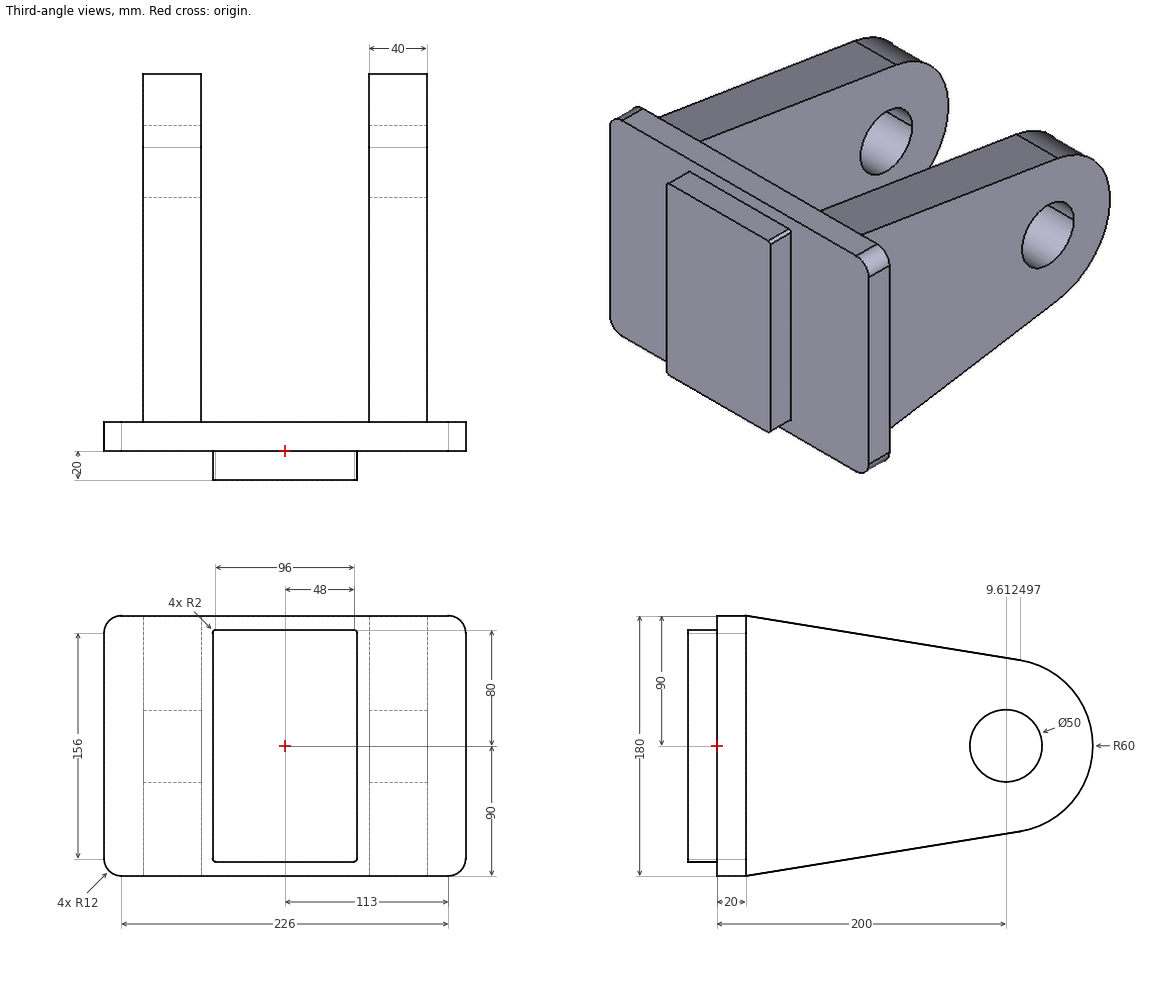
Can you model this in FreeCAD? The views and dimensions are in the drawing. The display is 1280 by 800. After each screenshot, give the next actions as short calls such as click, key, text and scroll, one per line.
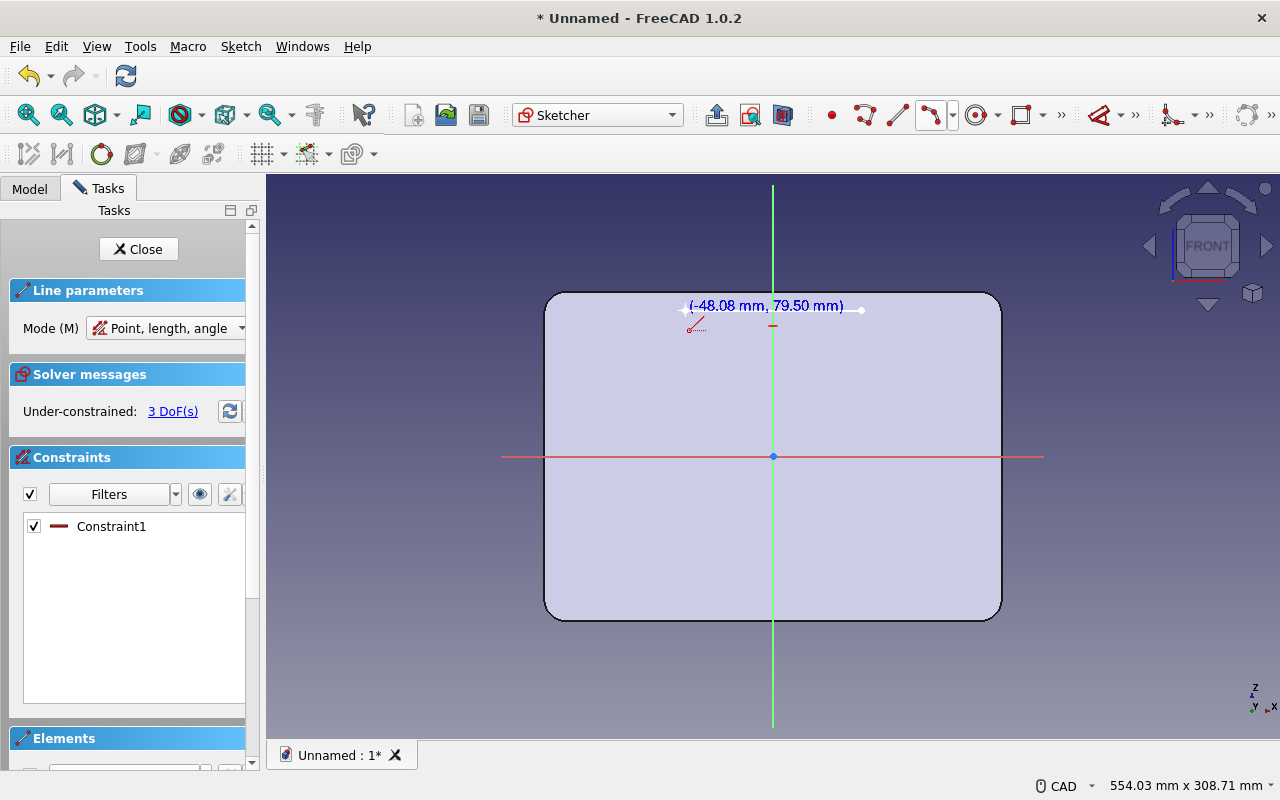
scroll(681, 314, up, 6)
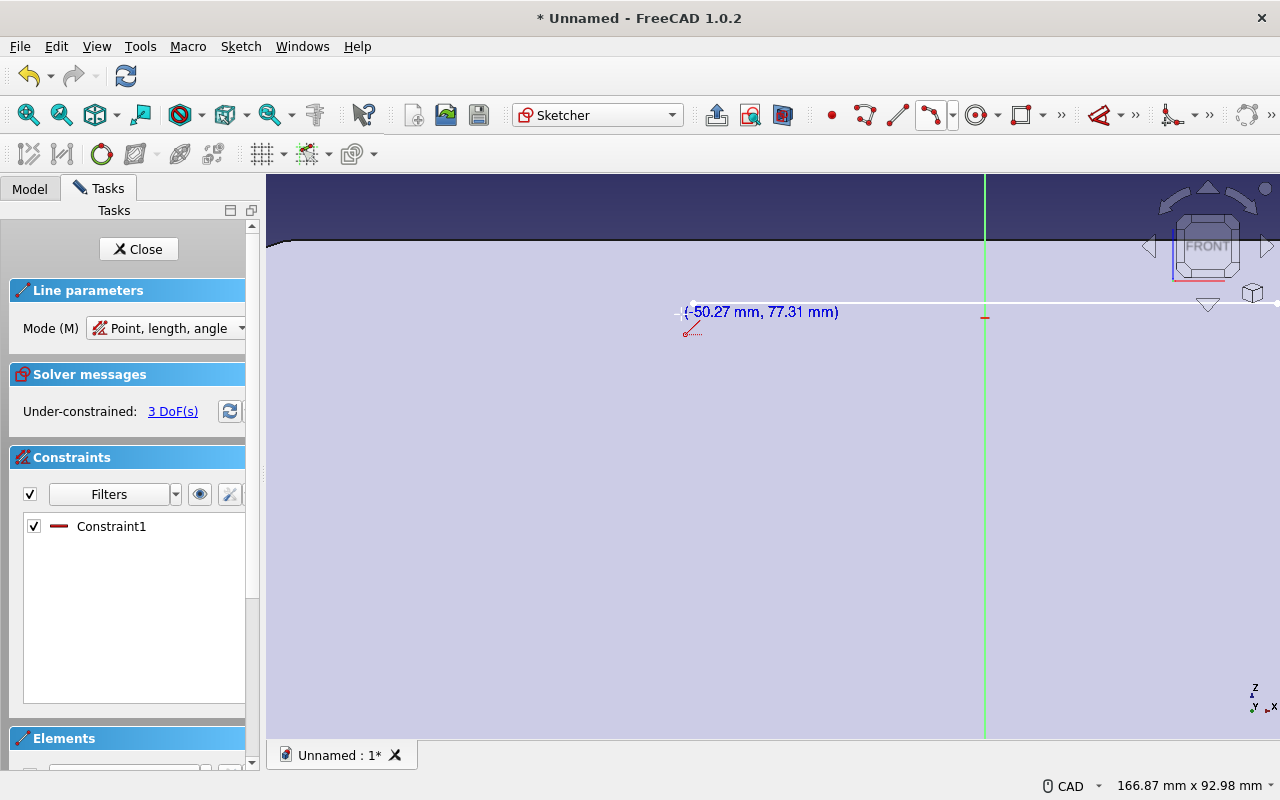
click(682, 313)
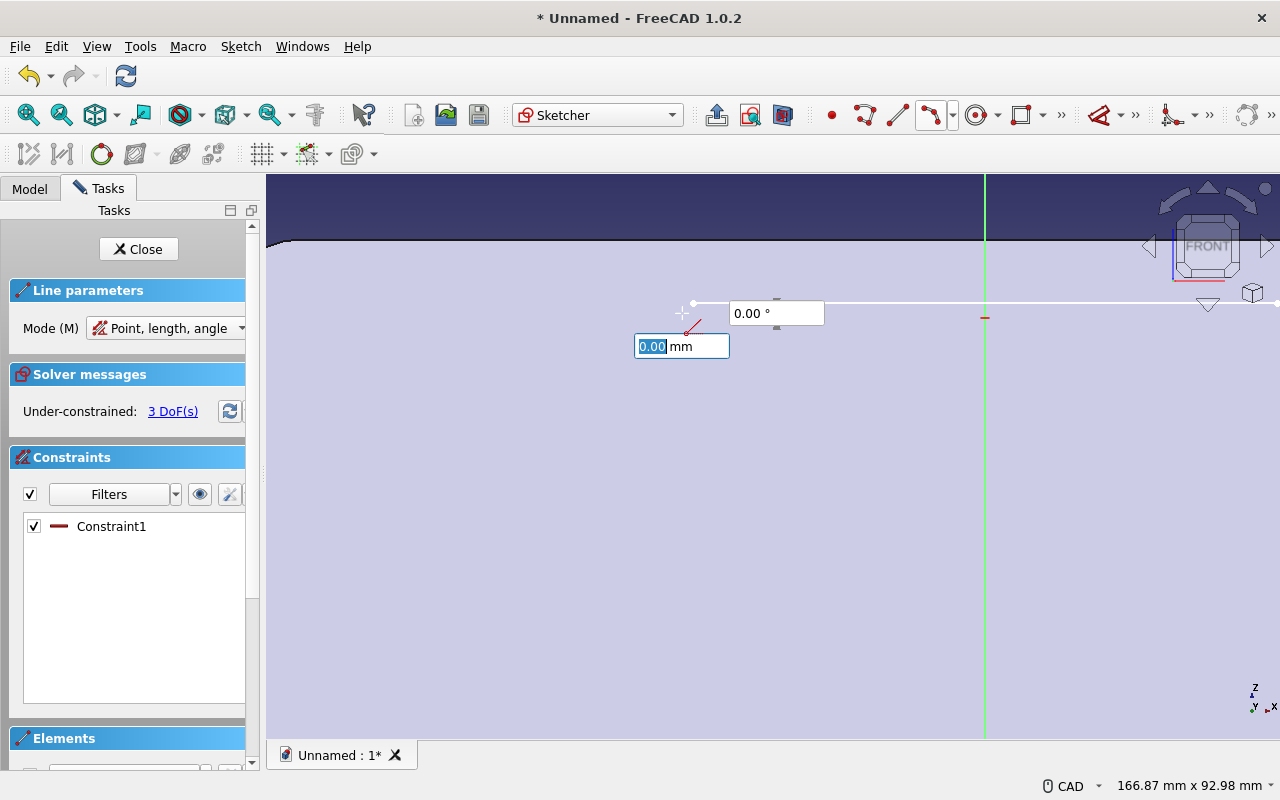
scroll(541, 264, down, 5)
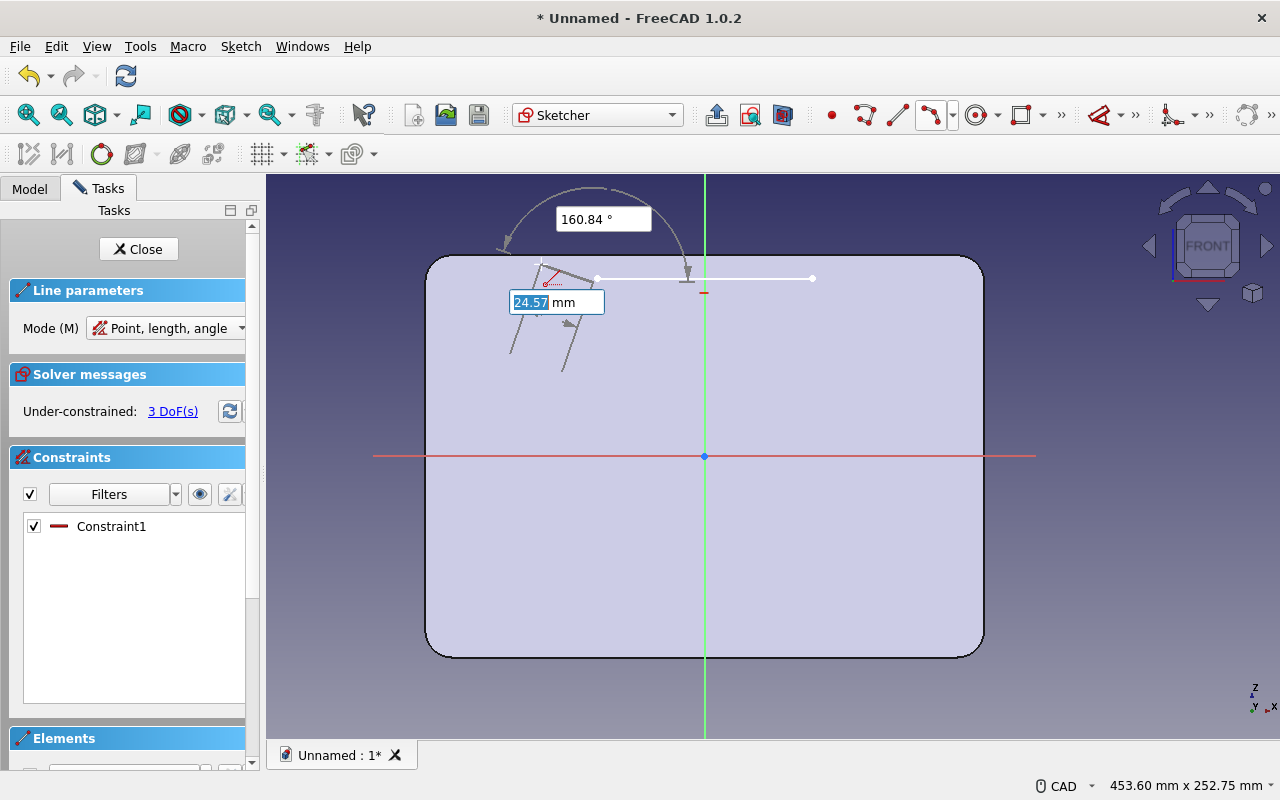
click(593, 631)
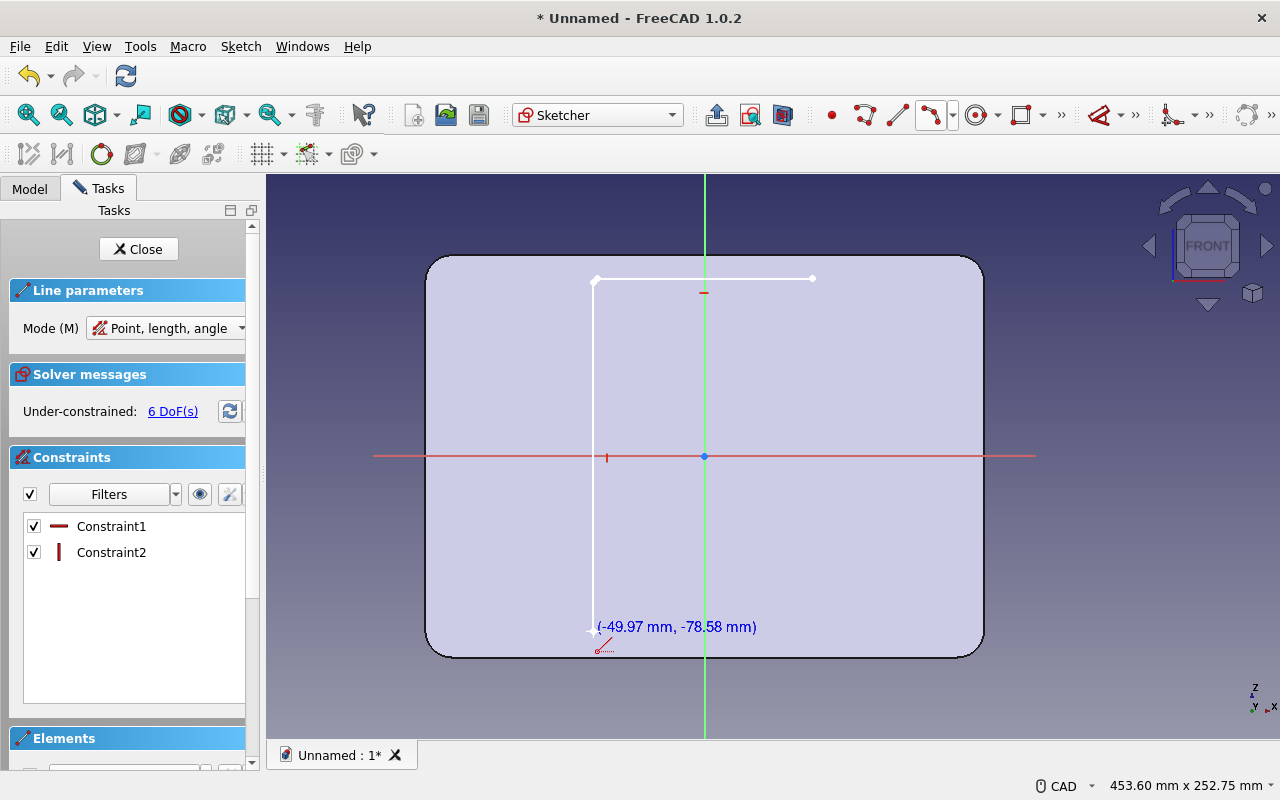
scroll(597, 635, up, 5)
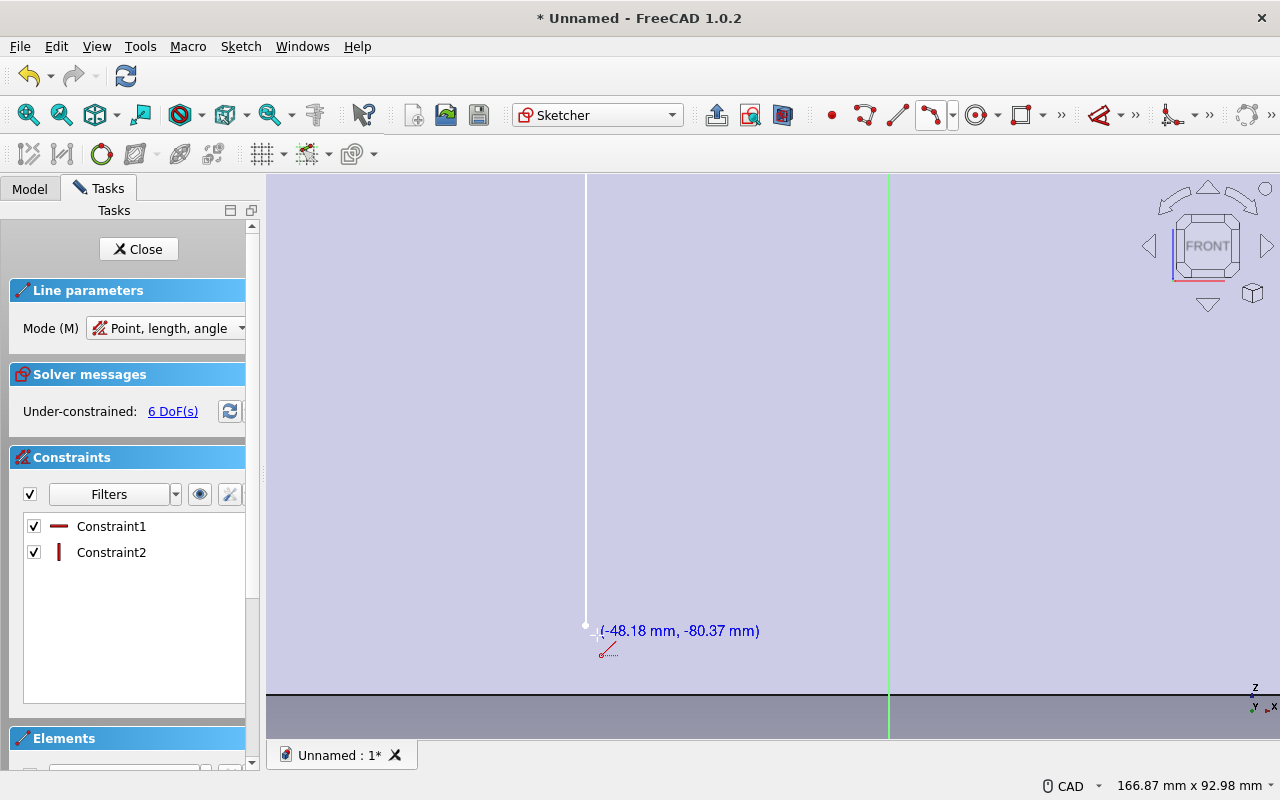
click(598, 634)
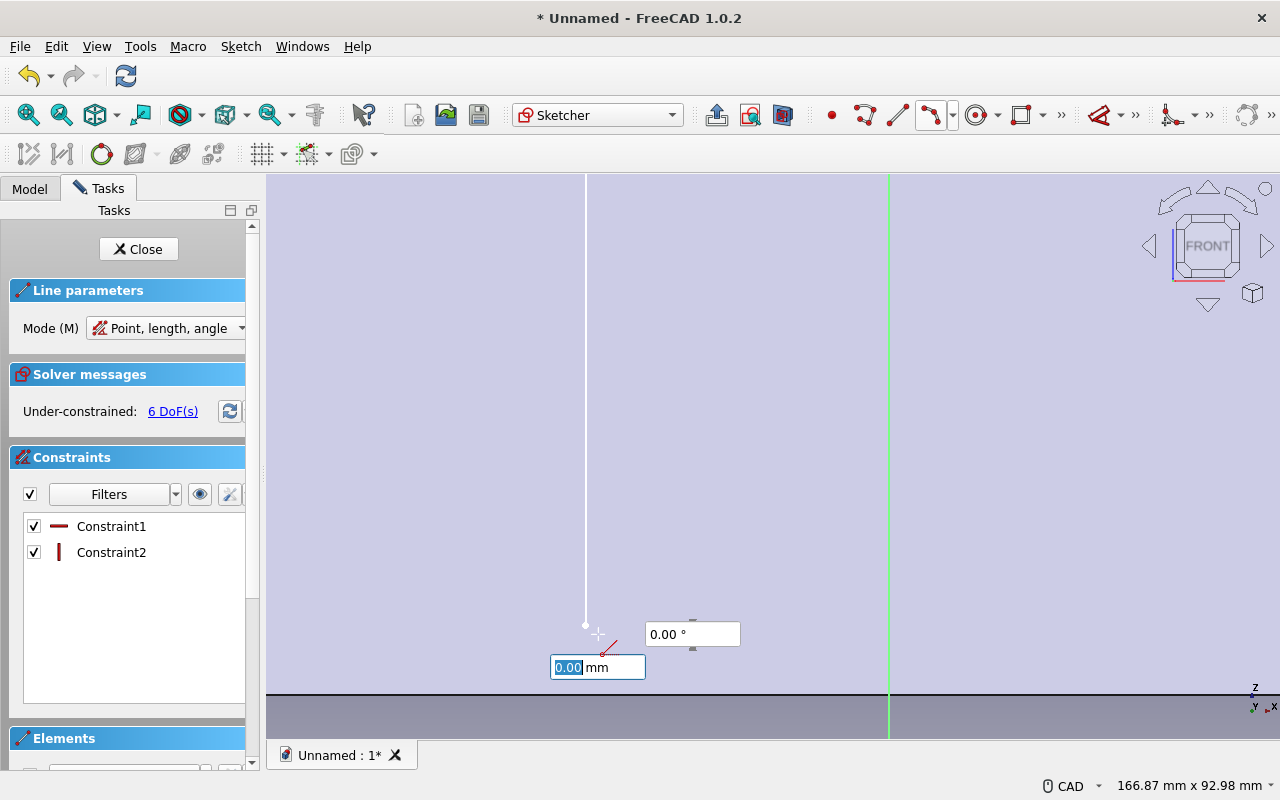
scroll(597, 636, down, 5)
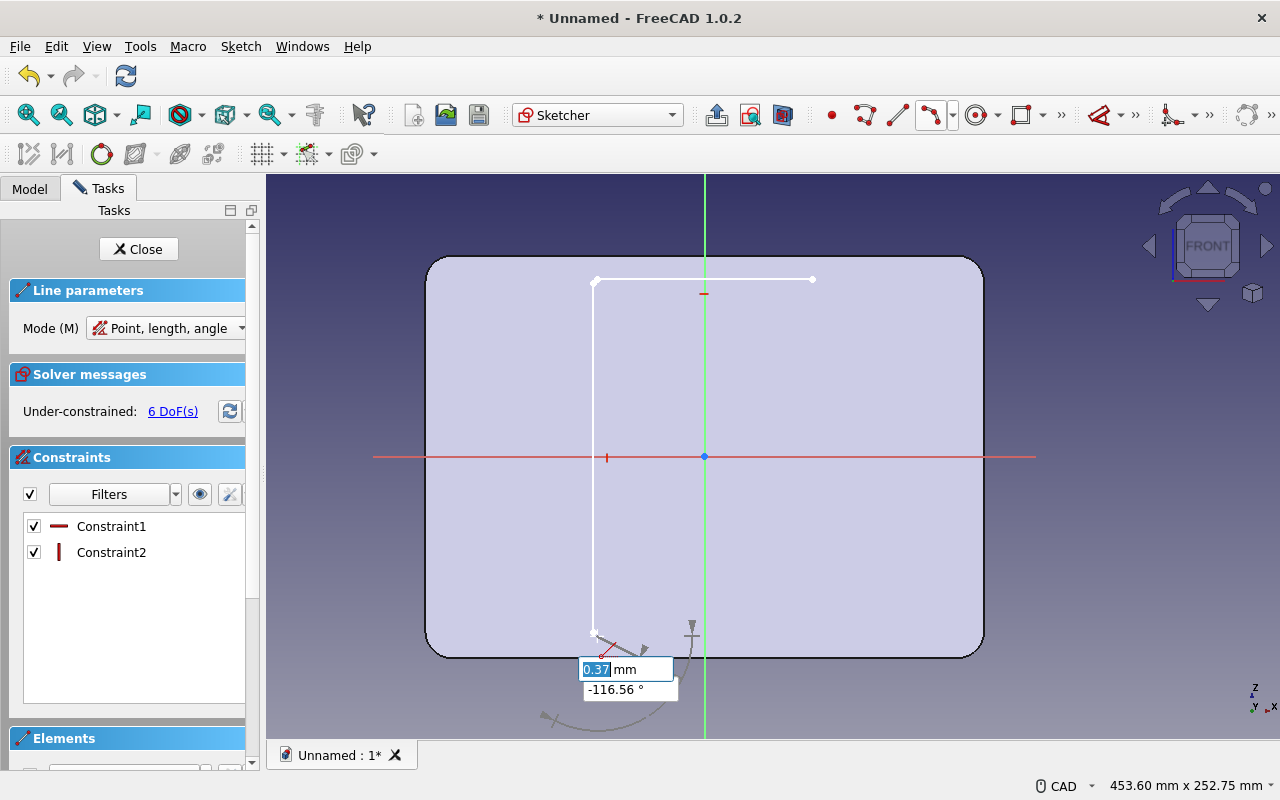
click(812, 636)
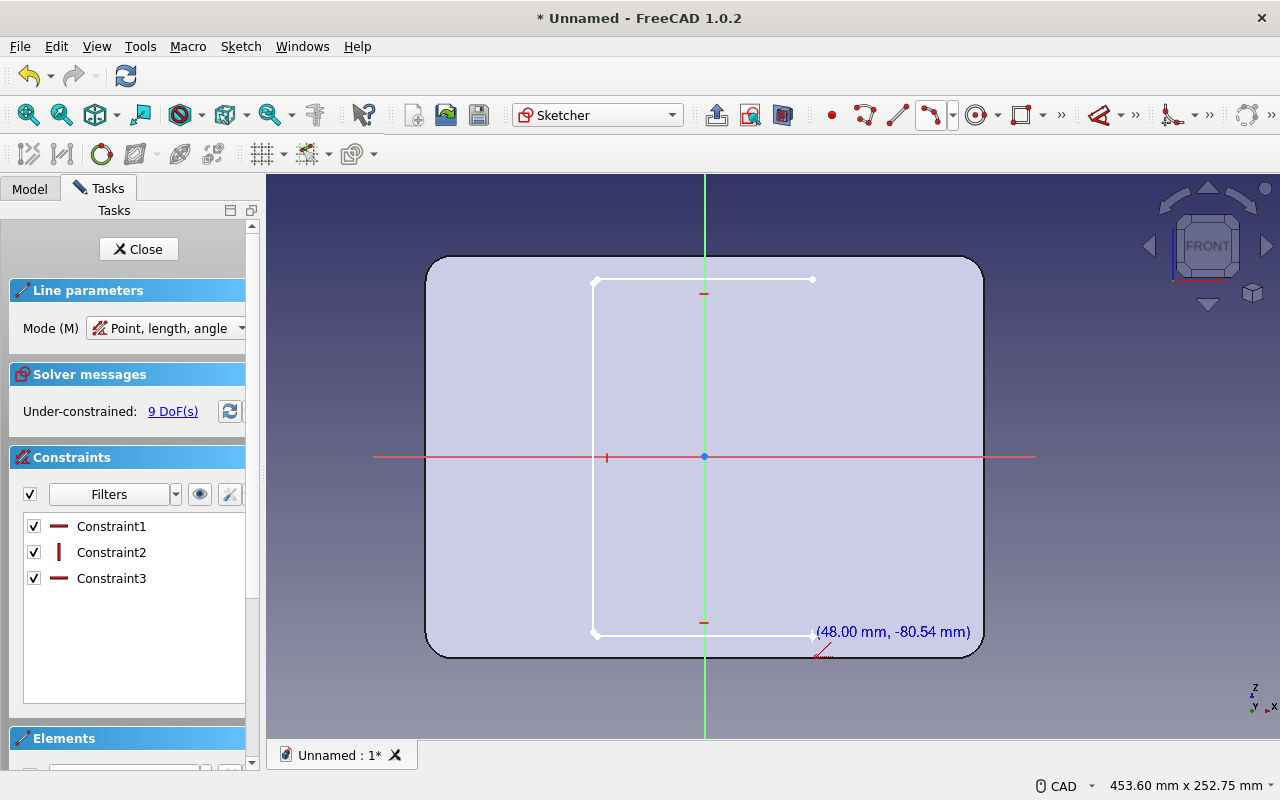
scroll(816, 631, up, 5)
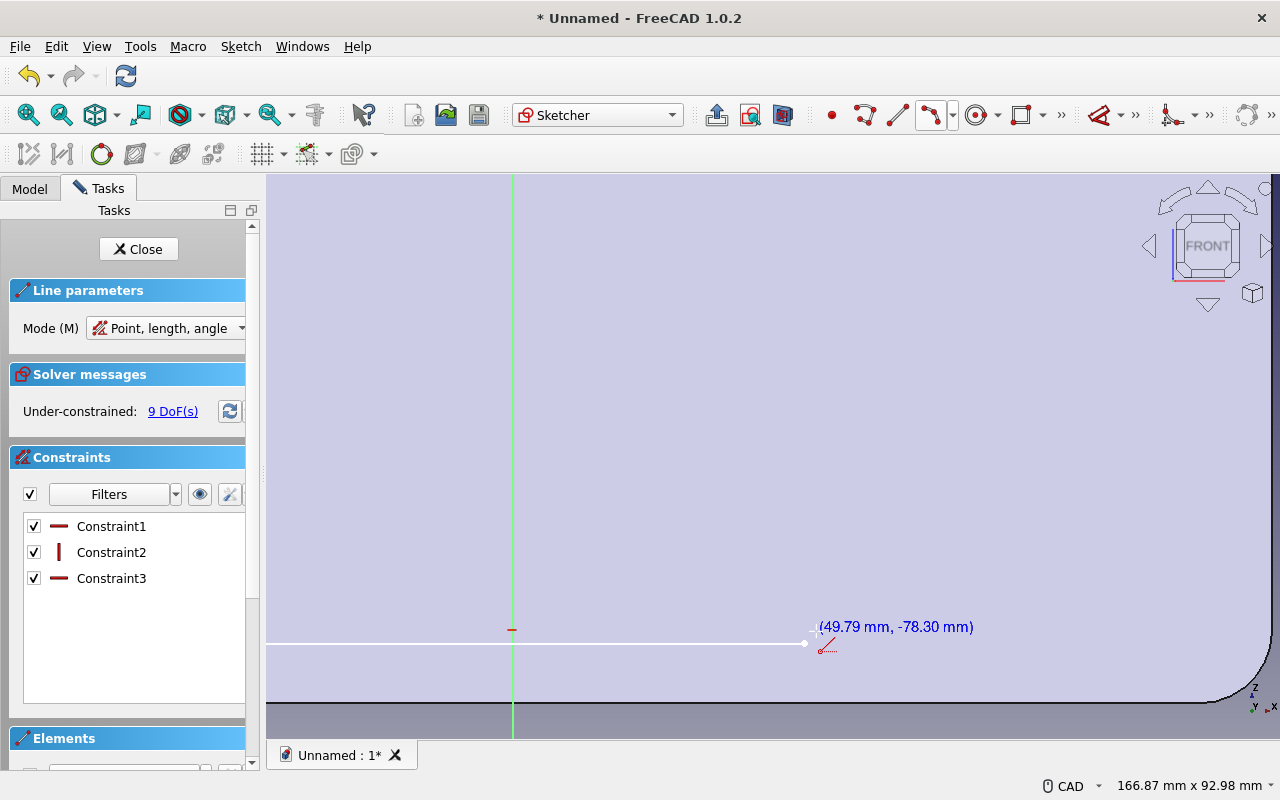
click(816, 631)